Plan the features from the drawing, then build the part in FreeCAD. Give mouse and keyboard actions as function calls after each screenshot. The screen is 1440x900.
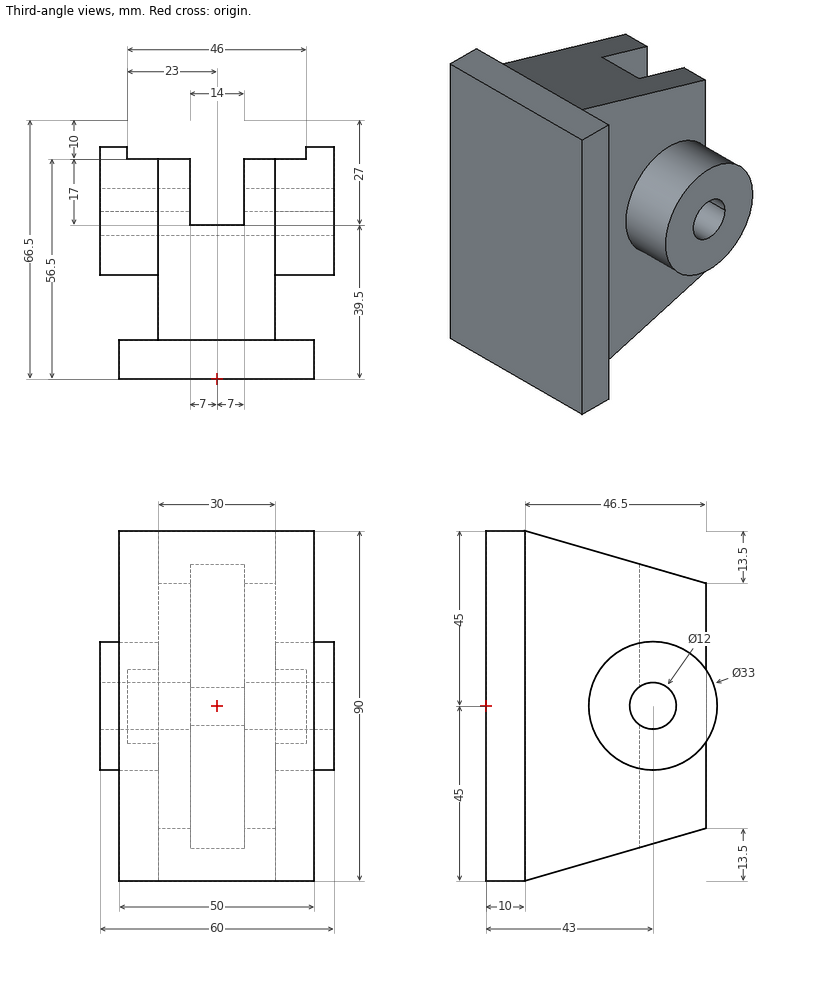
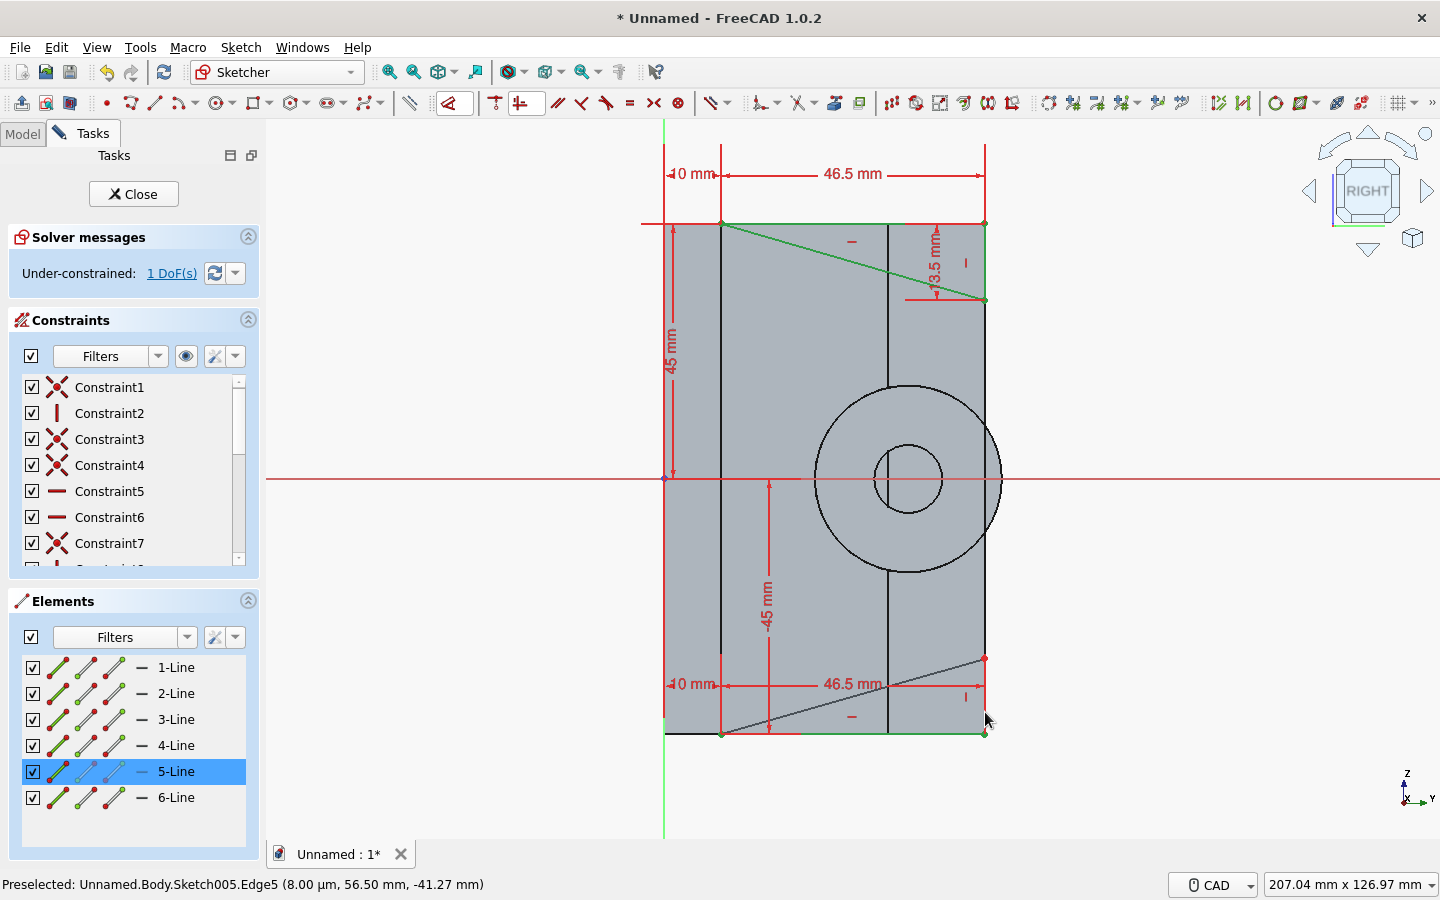
key(i)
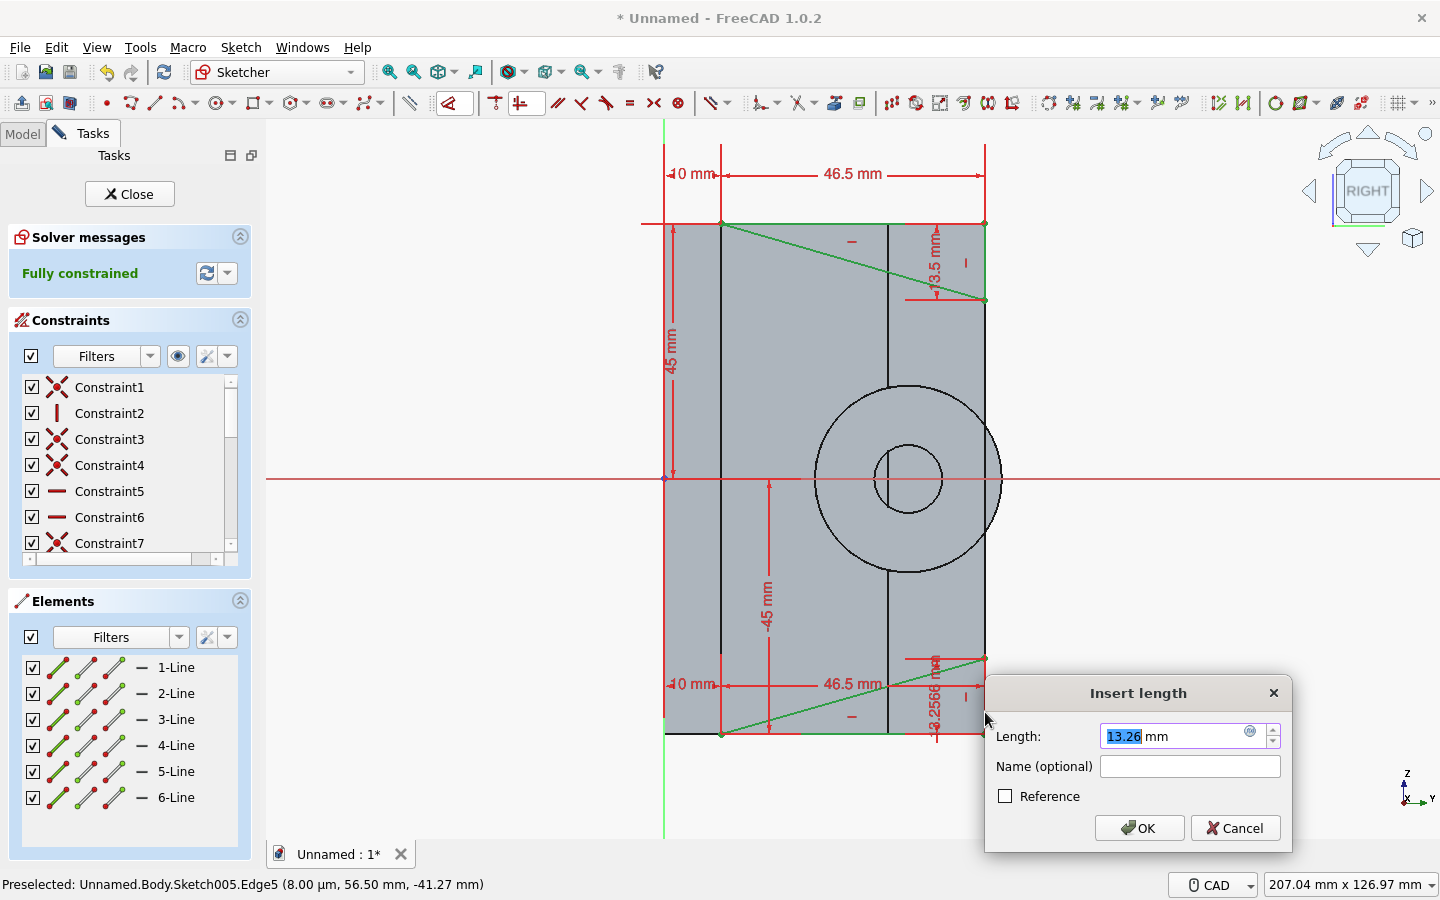
text(13.5)
key(Return)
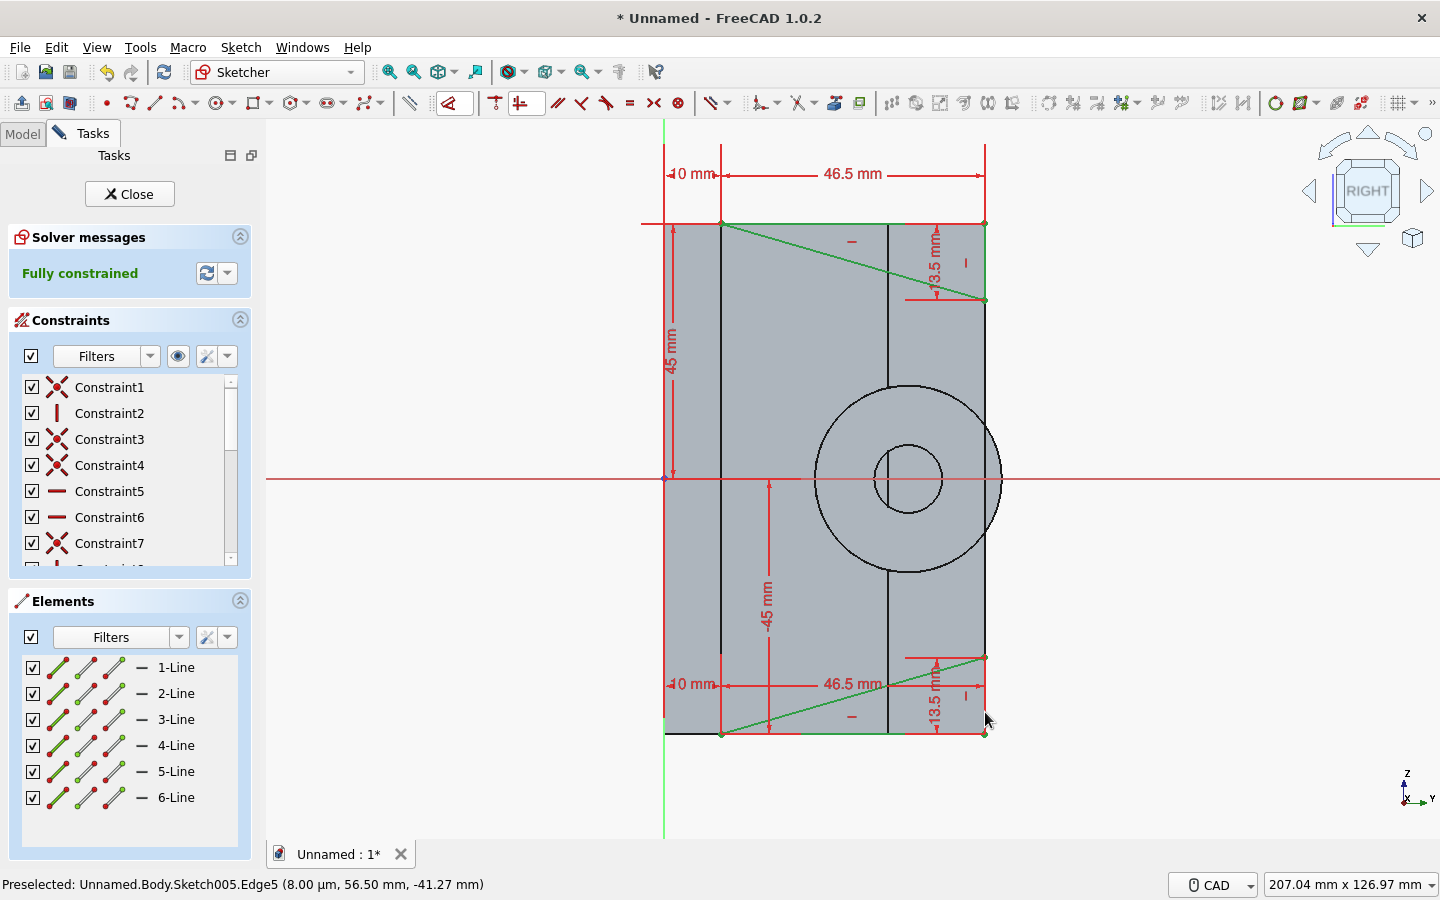
click(130, 194)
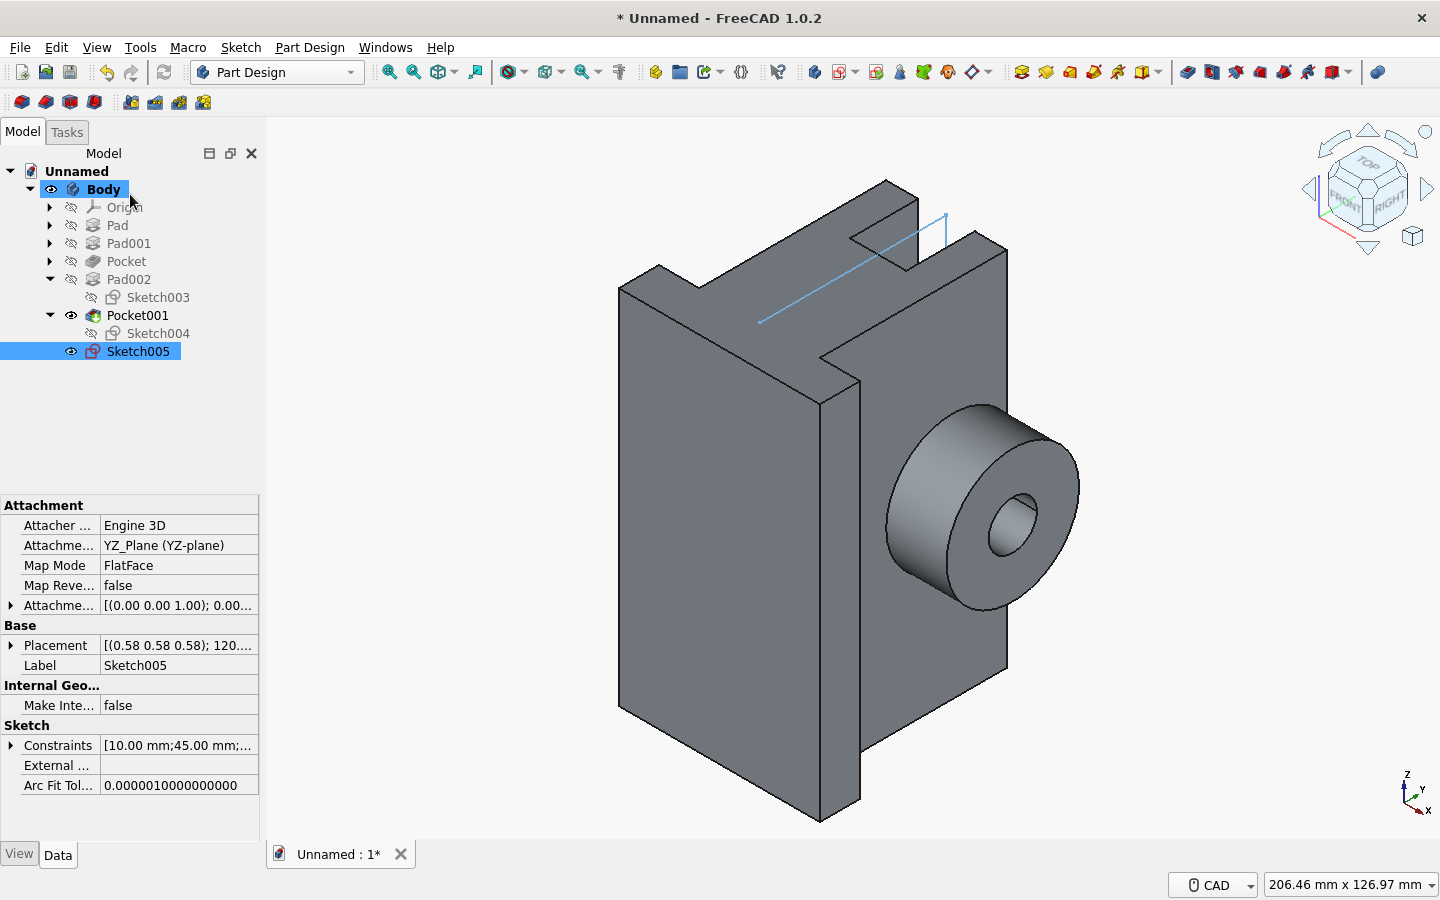
click(1188, 72)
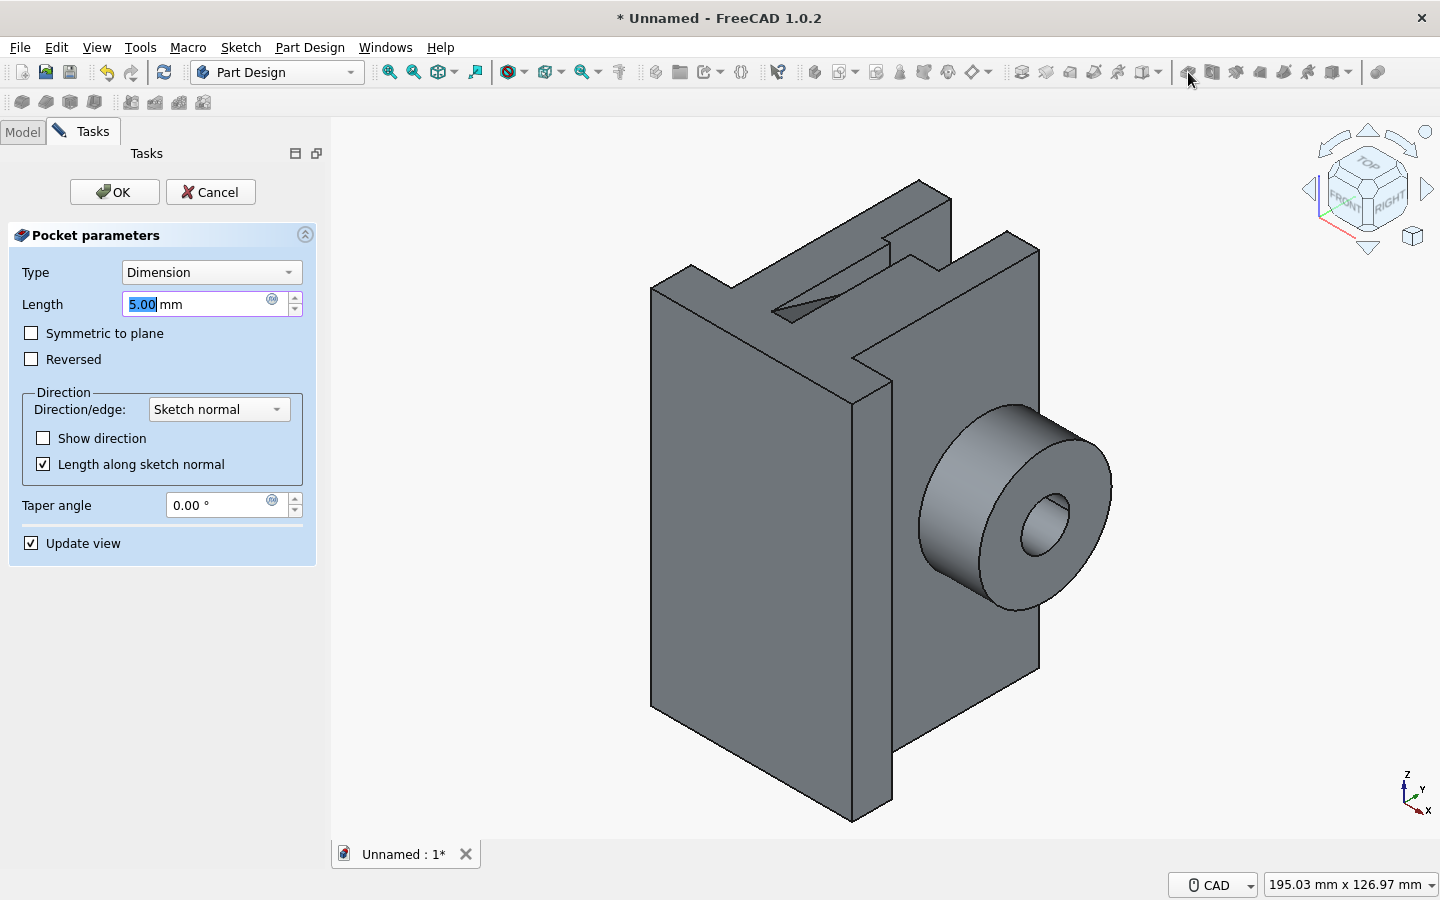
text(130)
key(Tab)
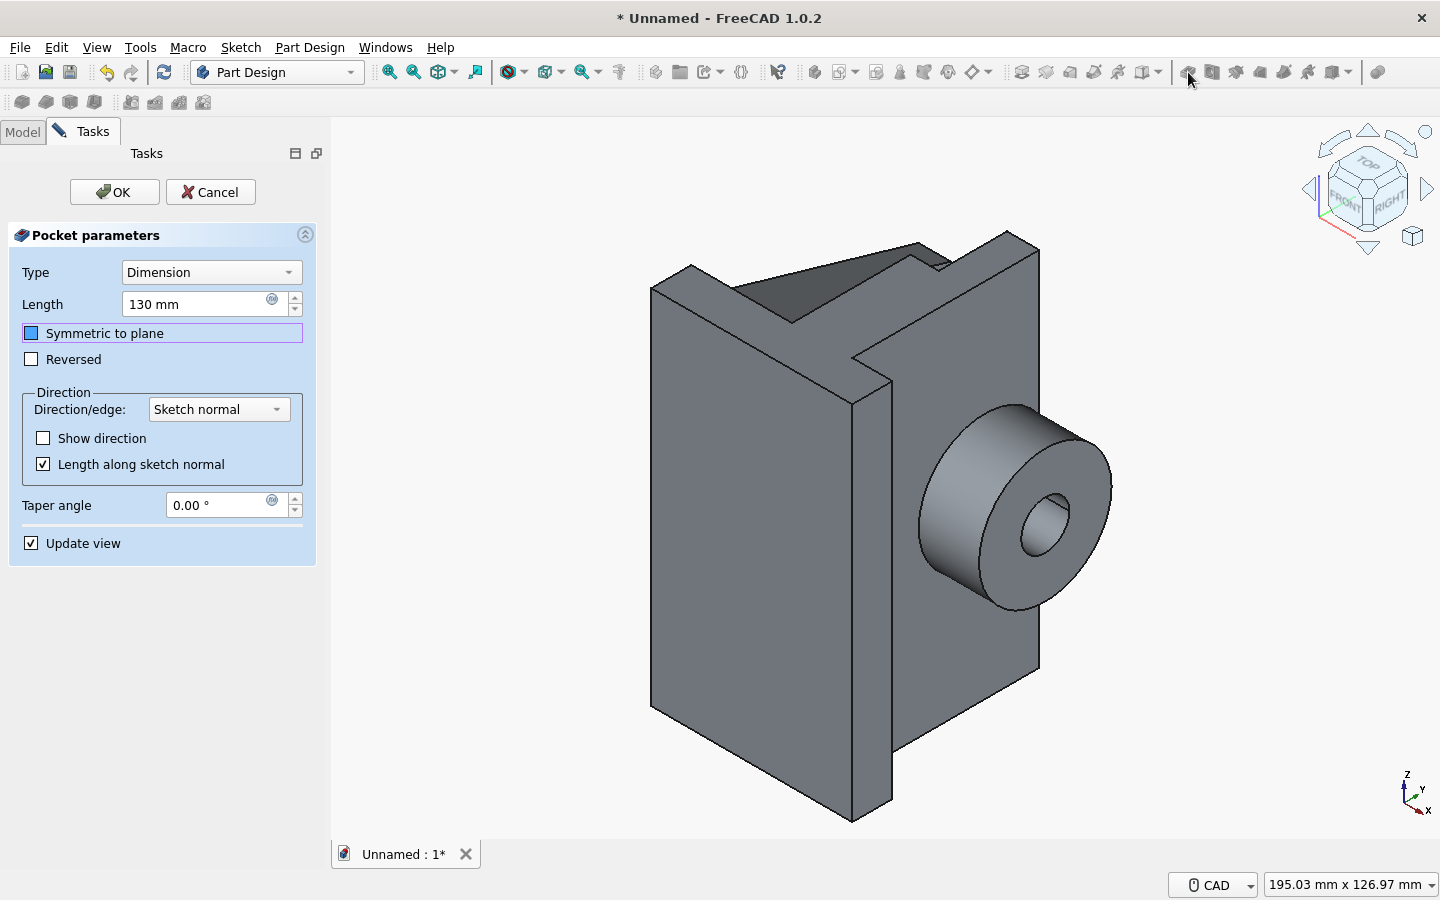
click(30, 333)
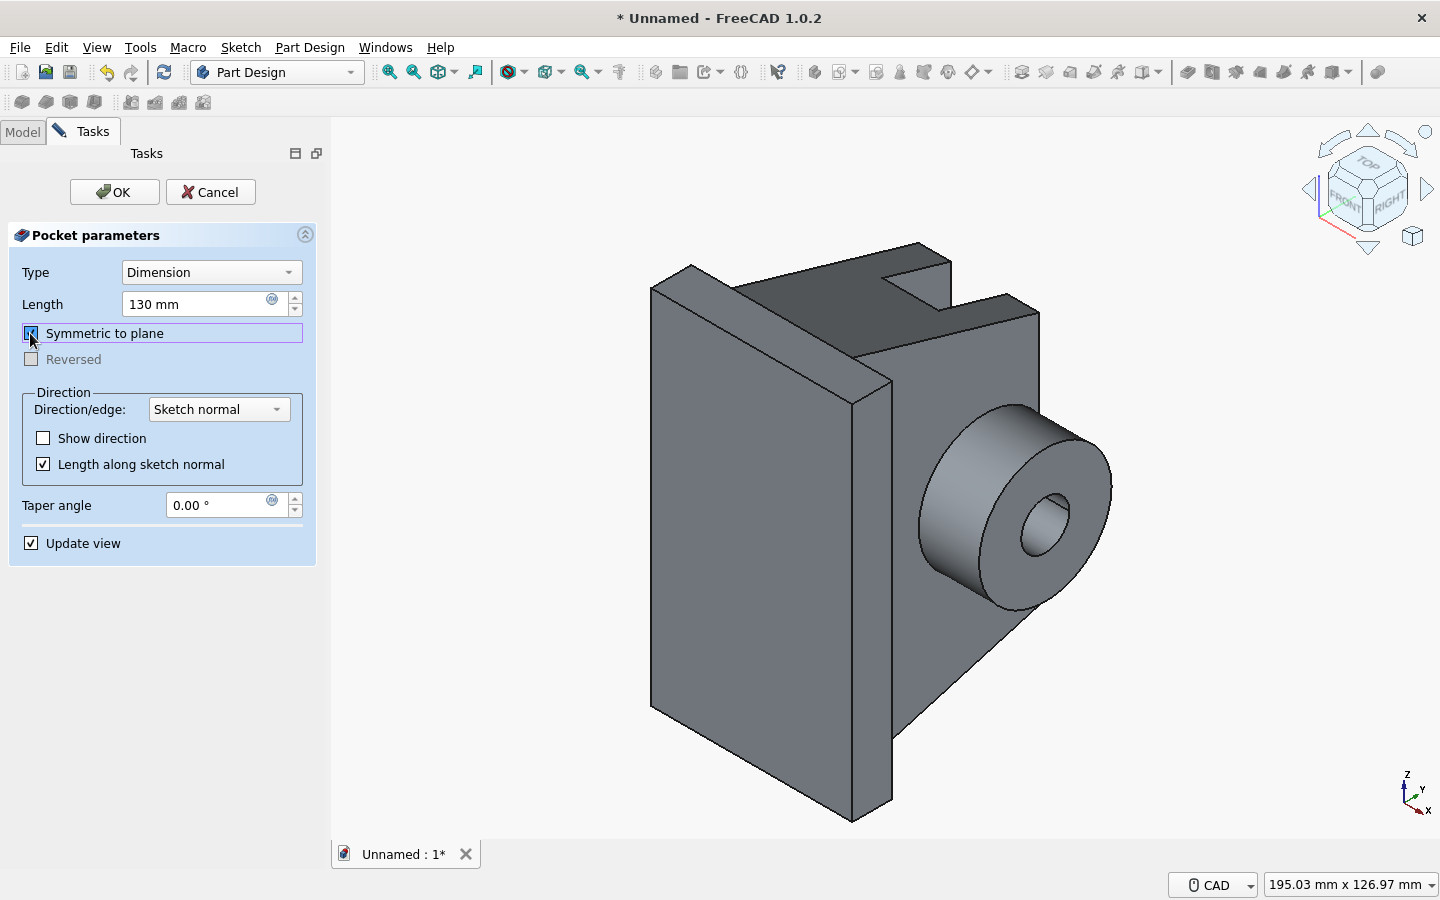
click(115, 192)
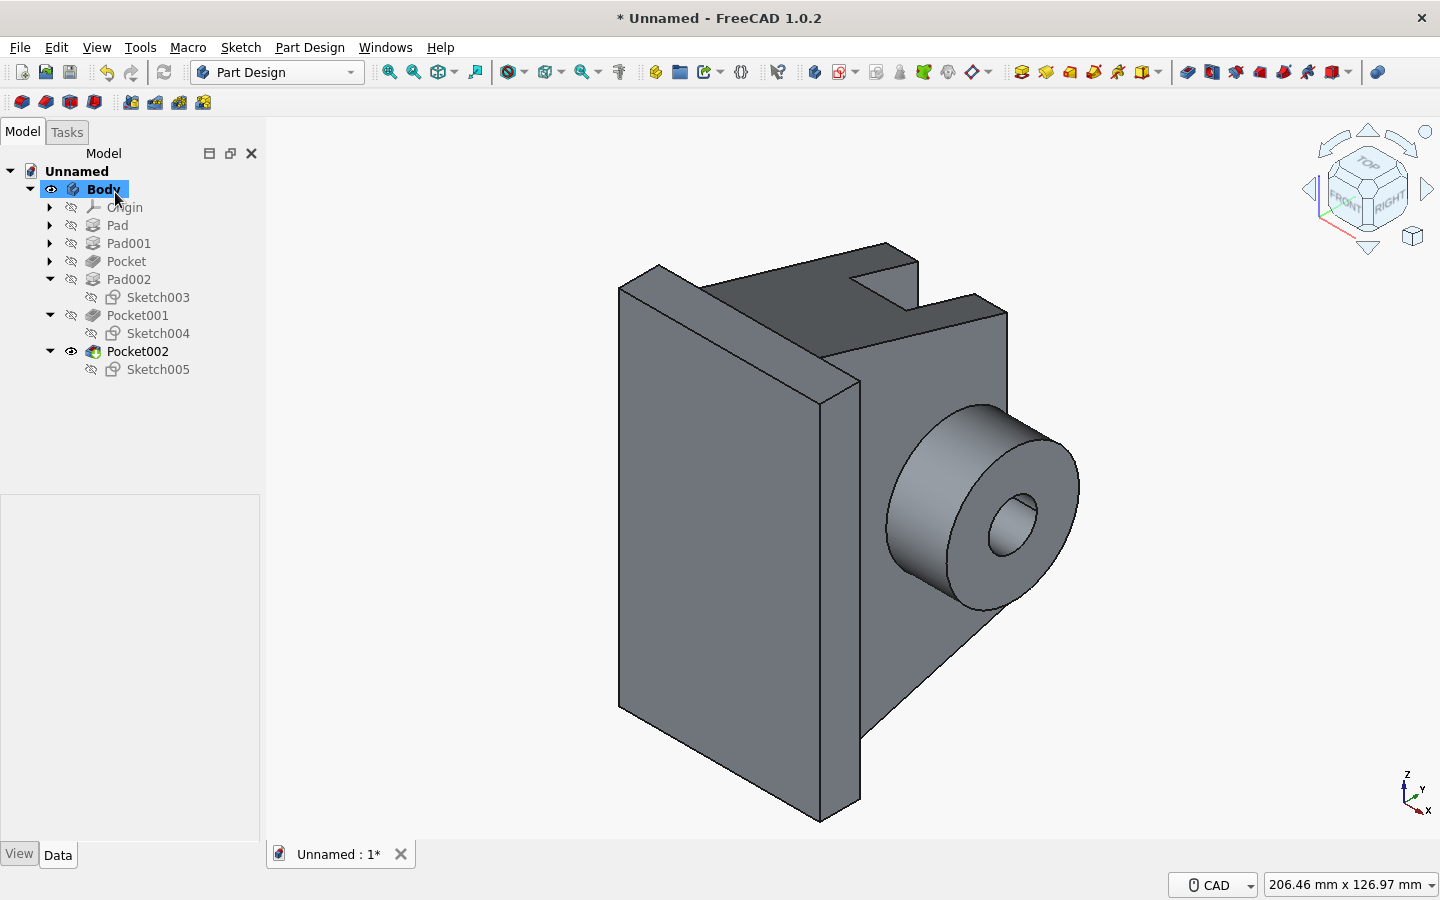
key(6)